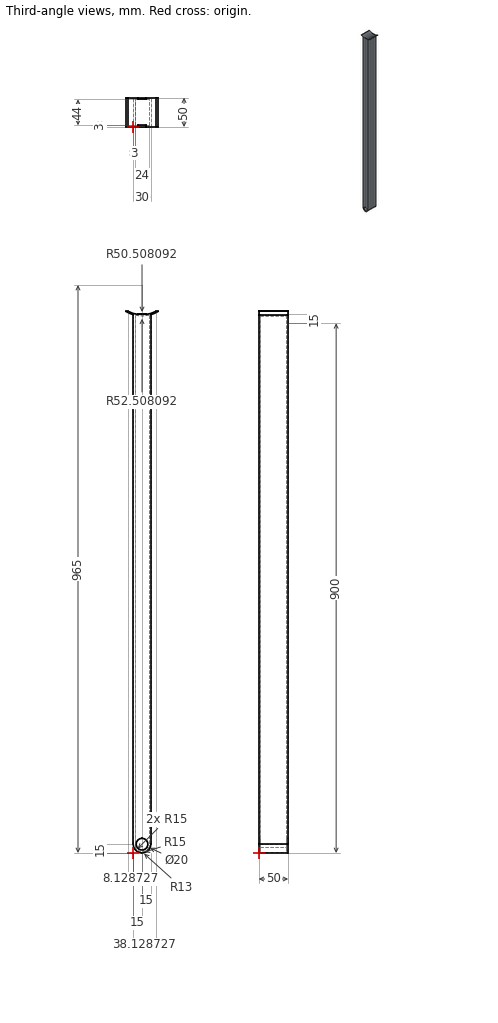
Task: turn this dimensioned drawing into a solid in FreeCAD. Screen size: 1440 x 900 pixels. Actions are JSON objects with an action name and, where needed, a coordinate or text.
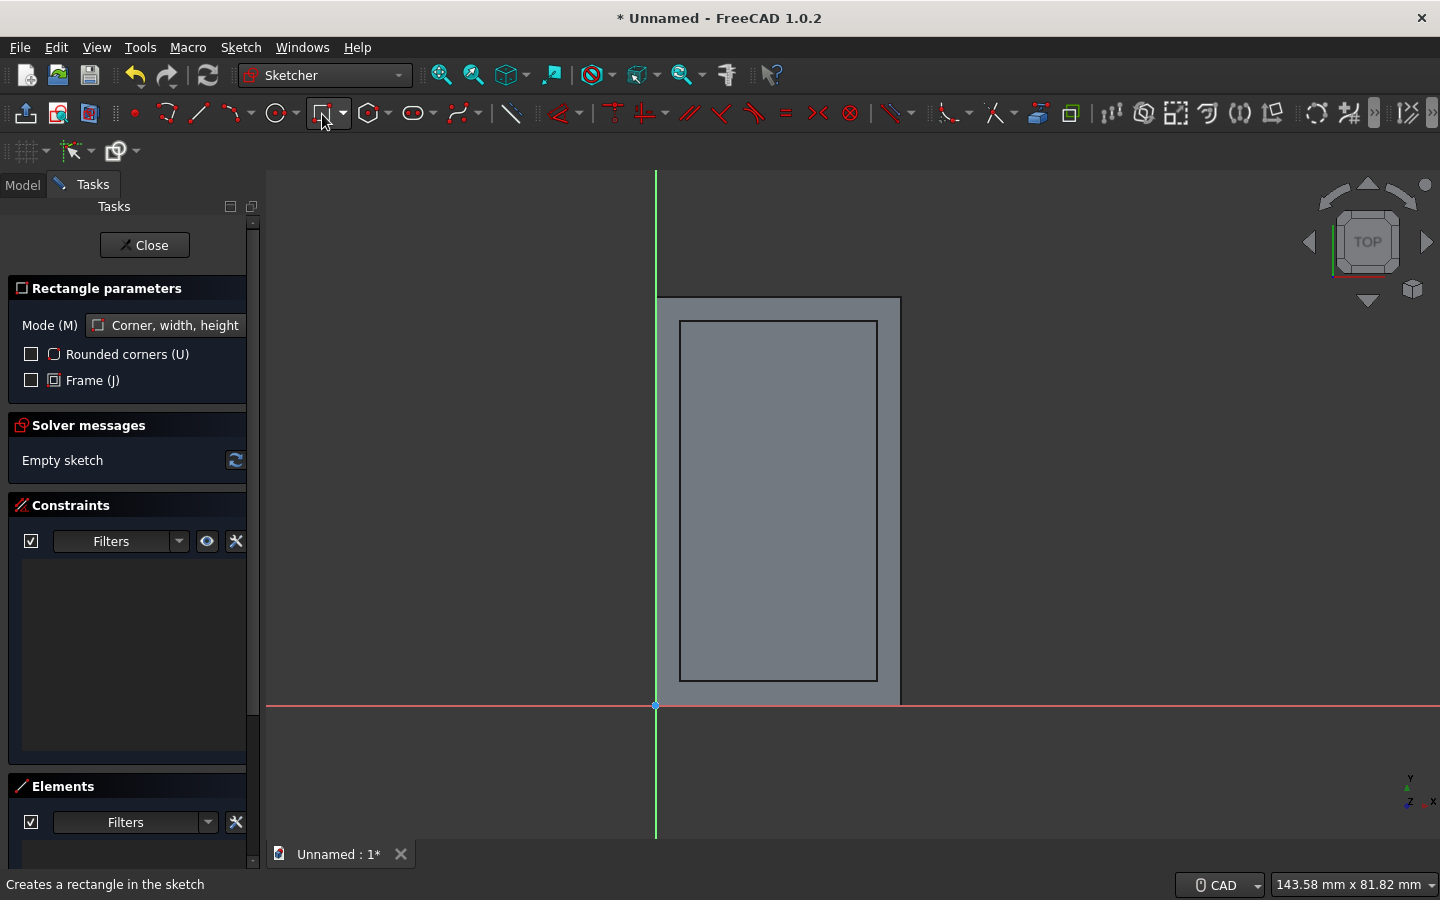
{"action": "left_click", "coordinate": [656, 706]}
{"action": "left_click", "coordinate": [901, 297]}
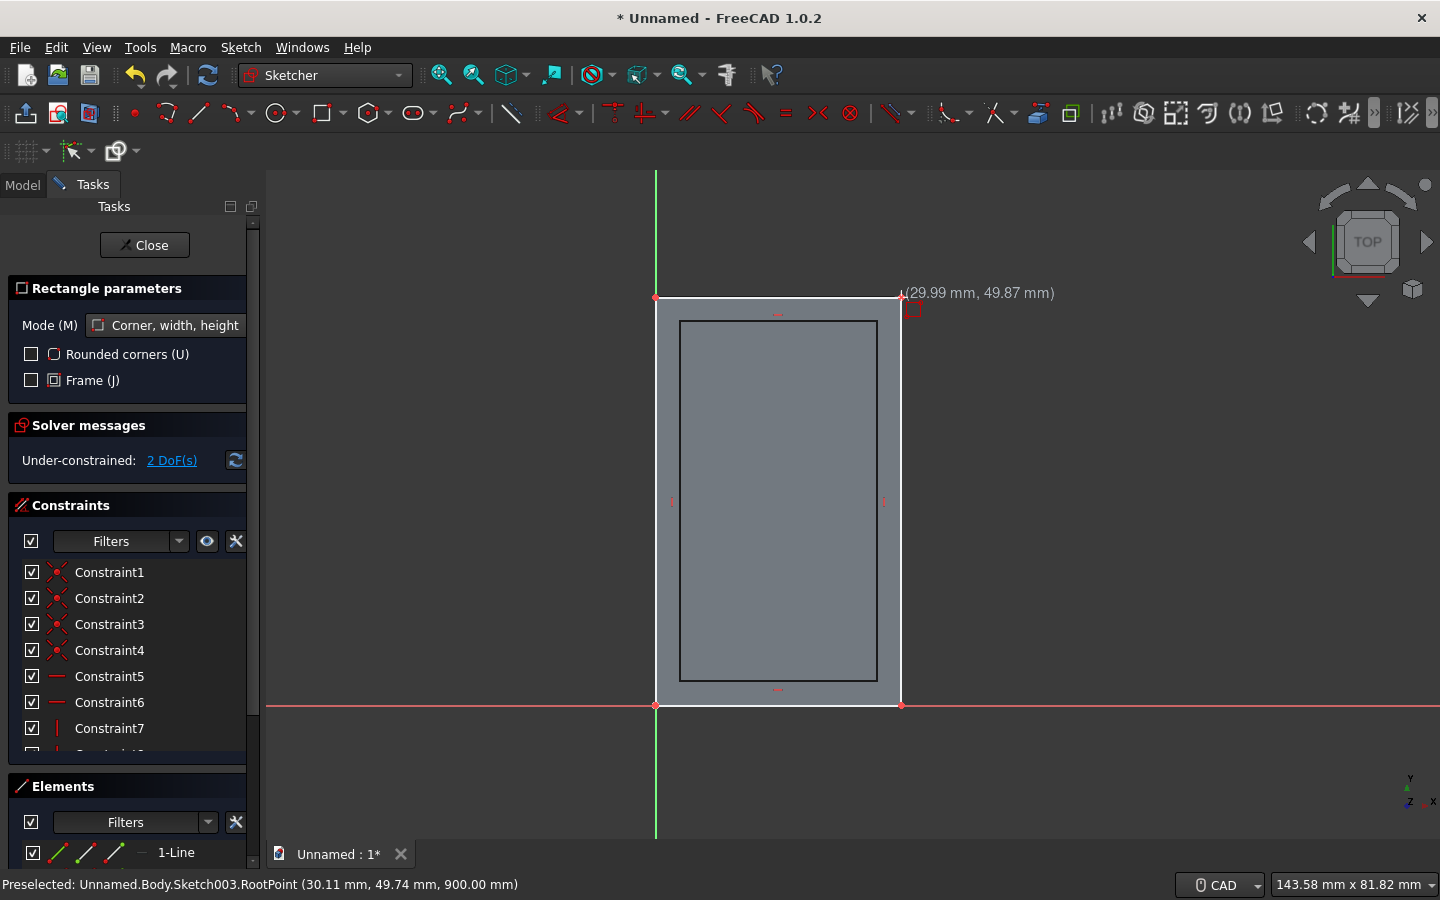
{"action": "left_click", "coordinate": [680, 321]}
{"action": "left_click", "coordinate": [877, 681]}
{"action": "key", "text": "Escape"}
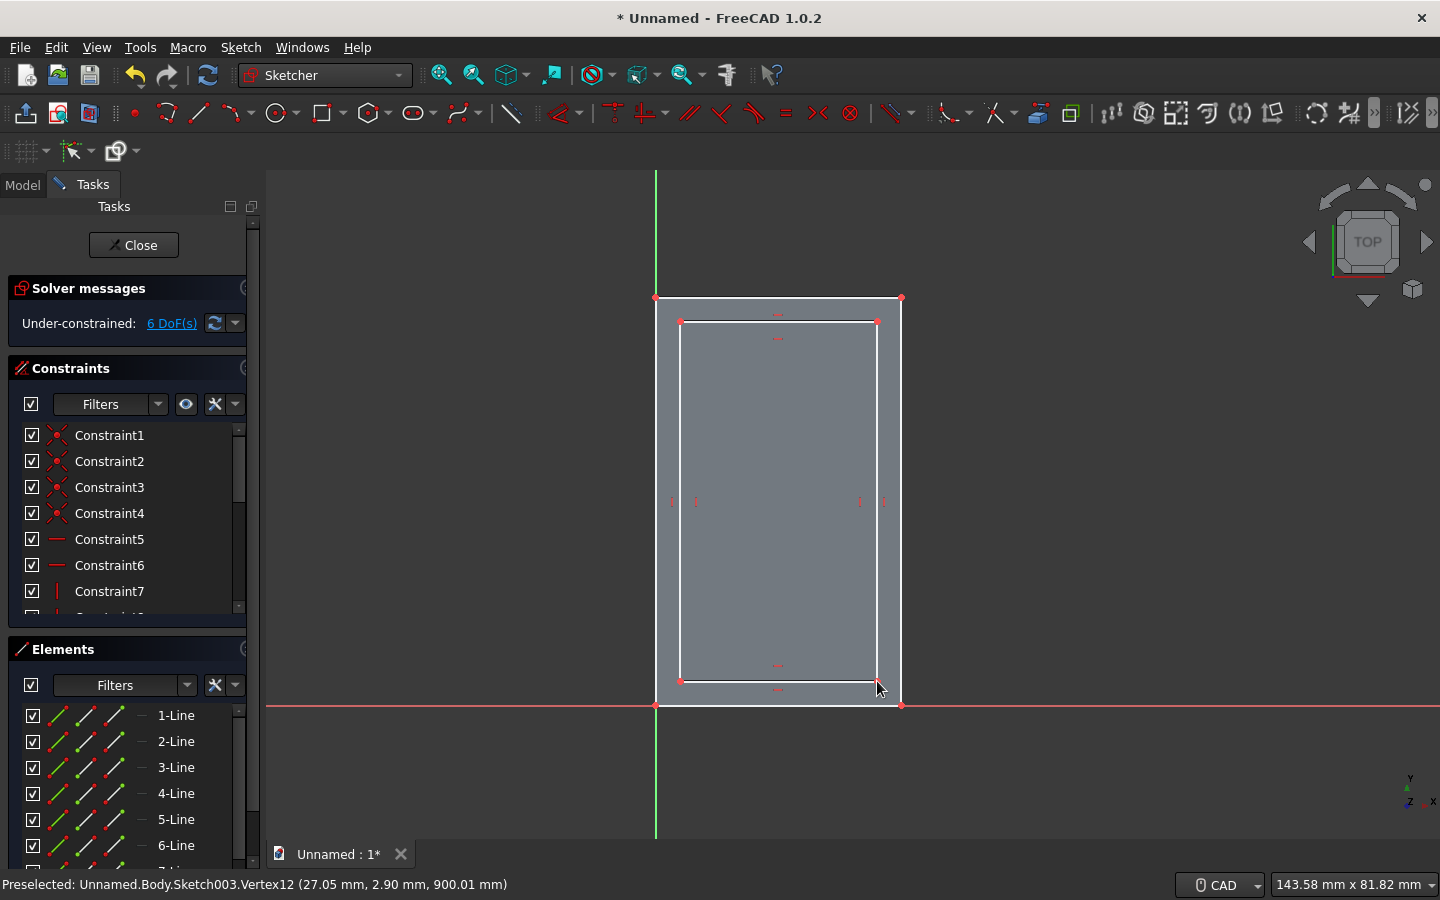
{"action": "left_click", "coordinate": [558, 114]}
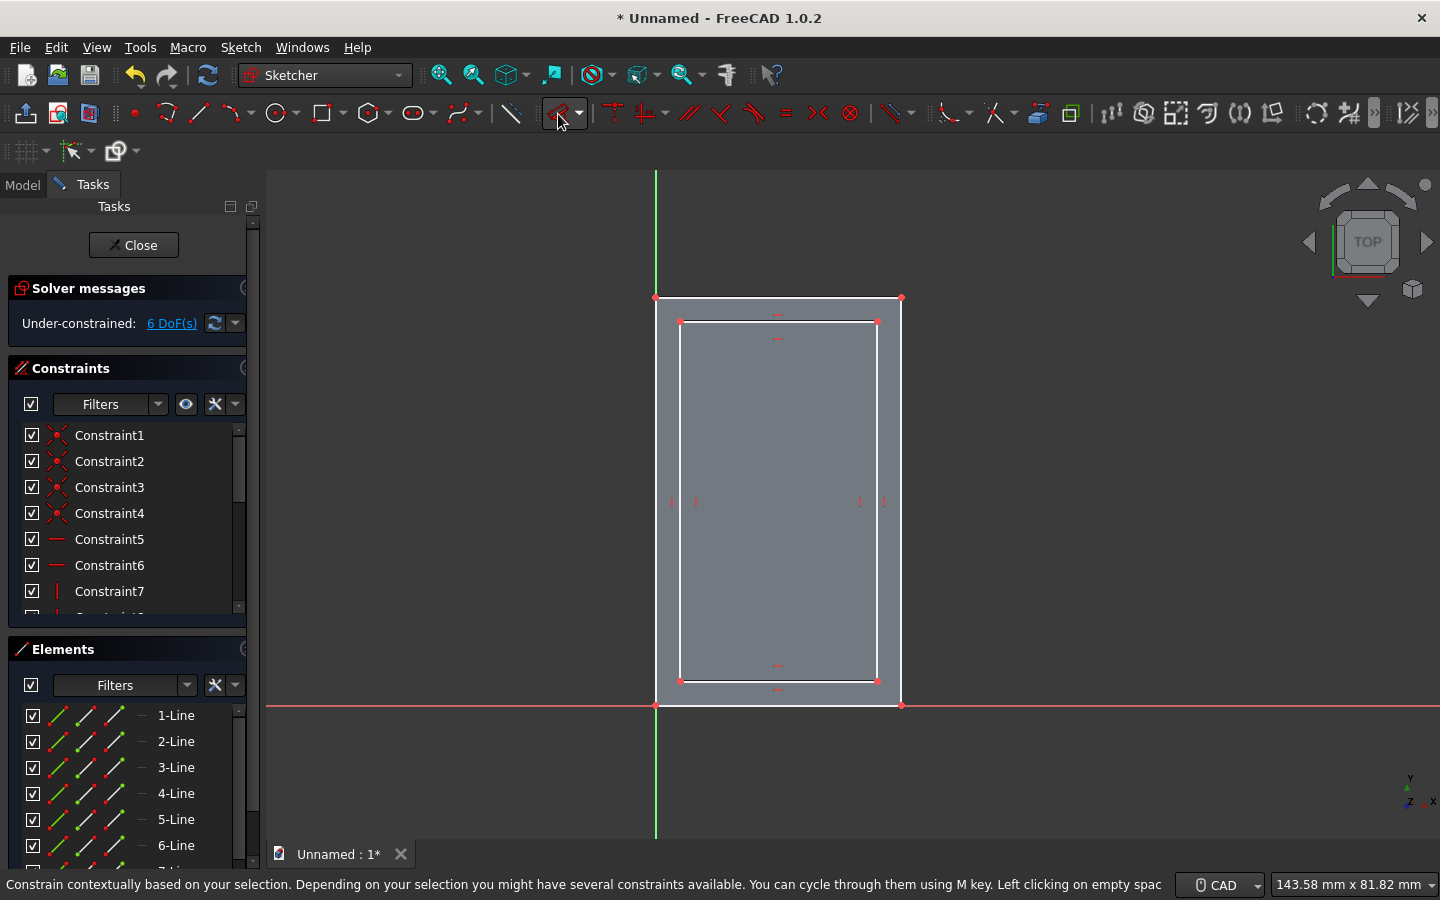
{"action": "left_click", "coordinate": [729, 706]}
{"action": "left_click", "coordinate": [778, 740]}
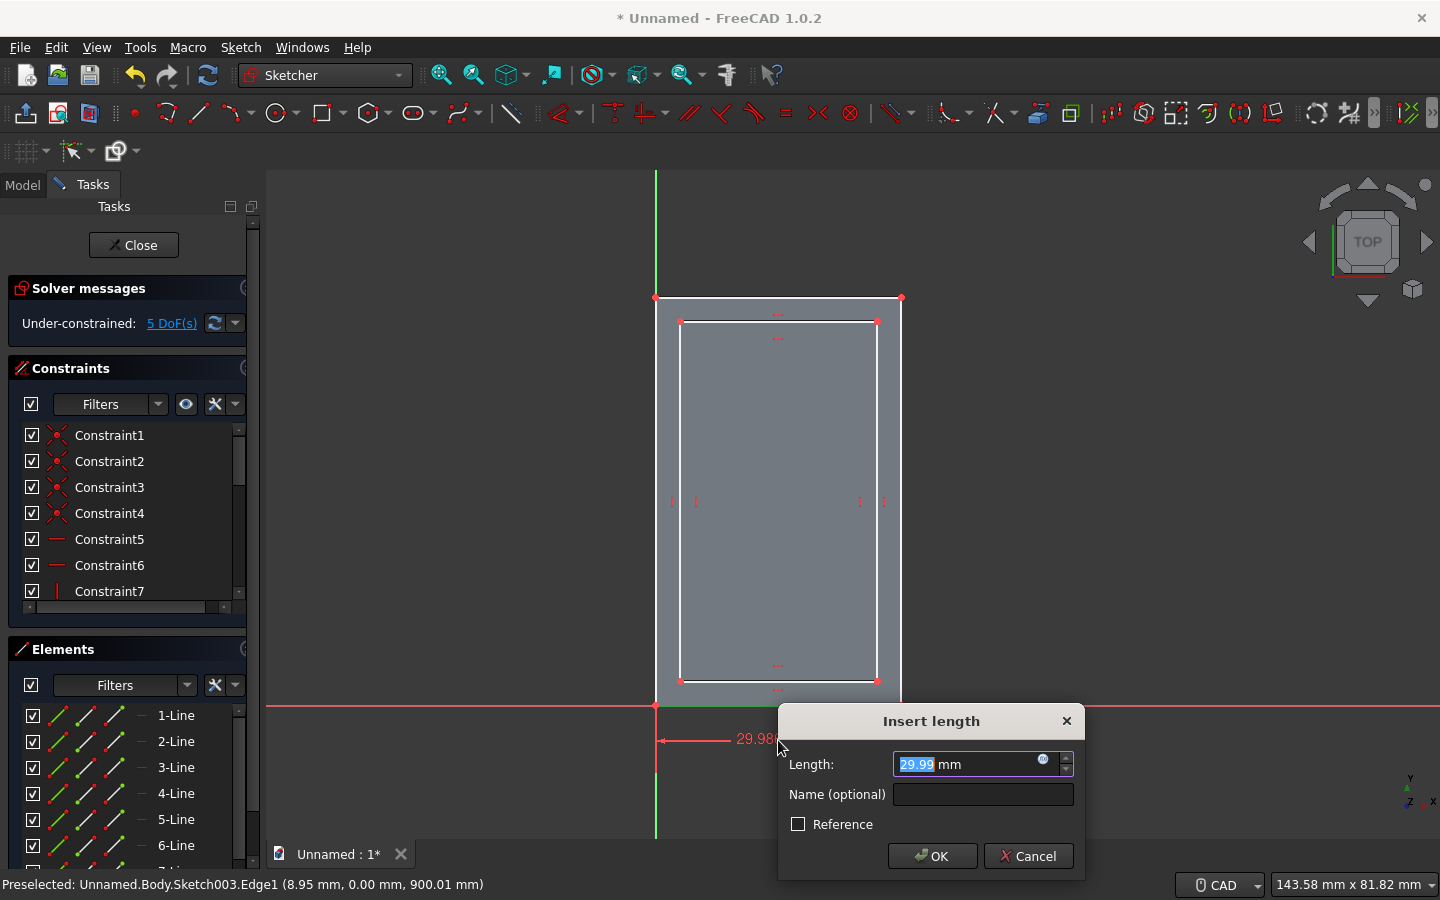
{"action": "type", "text": "30"}
{"action": "key", "text": "Return"}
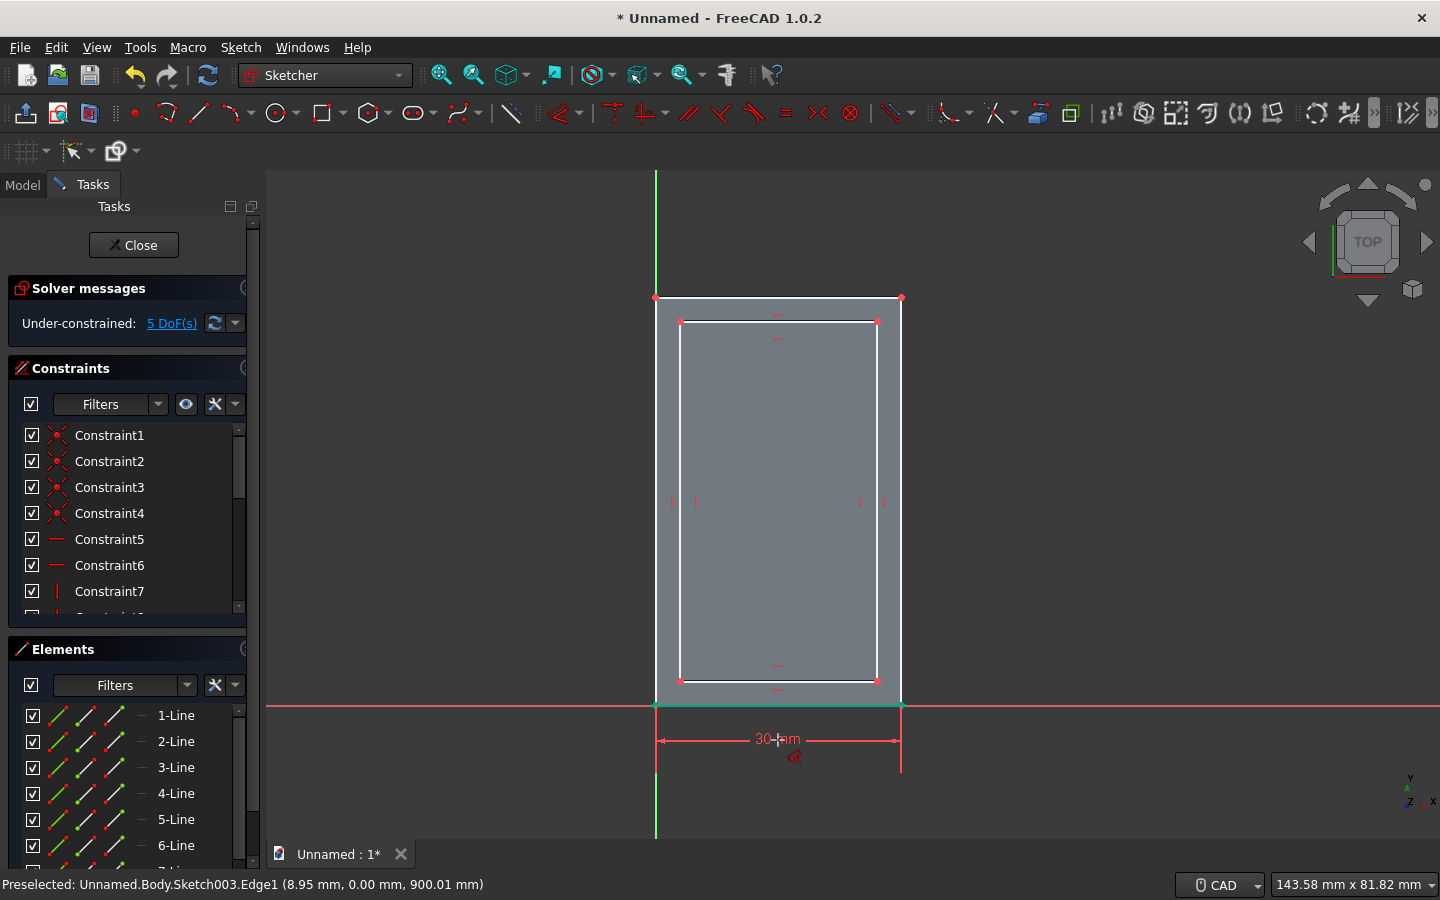
{"action": "left_click", "coordinate": [901, 583]}
{"action": "left_click", "coordinate": [935, 502]}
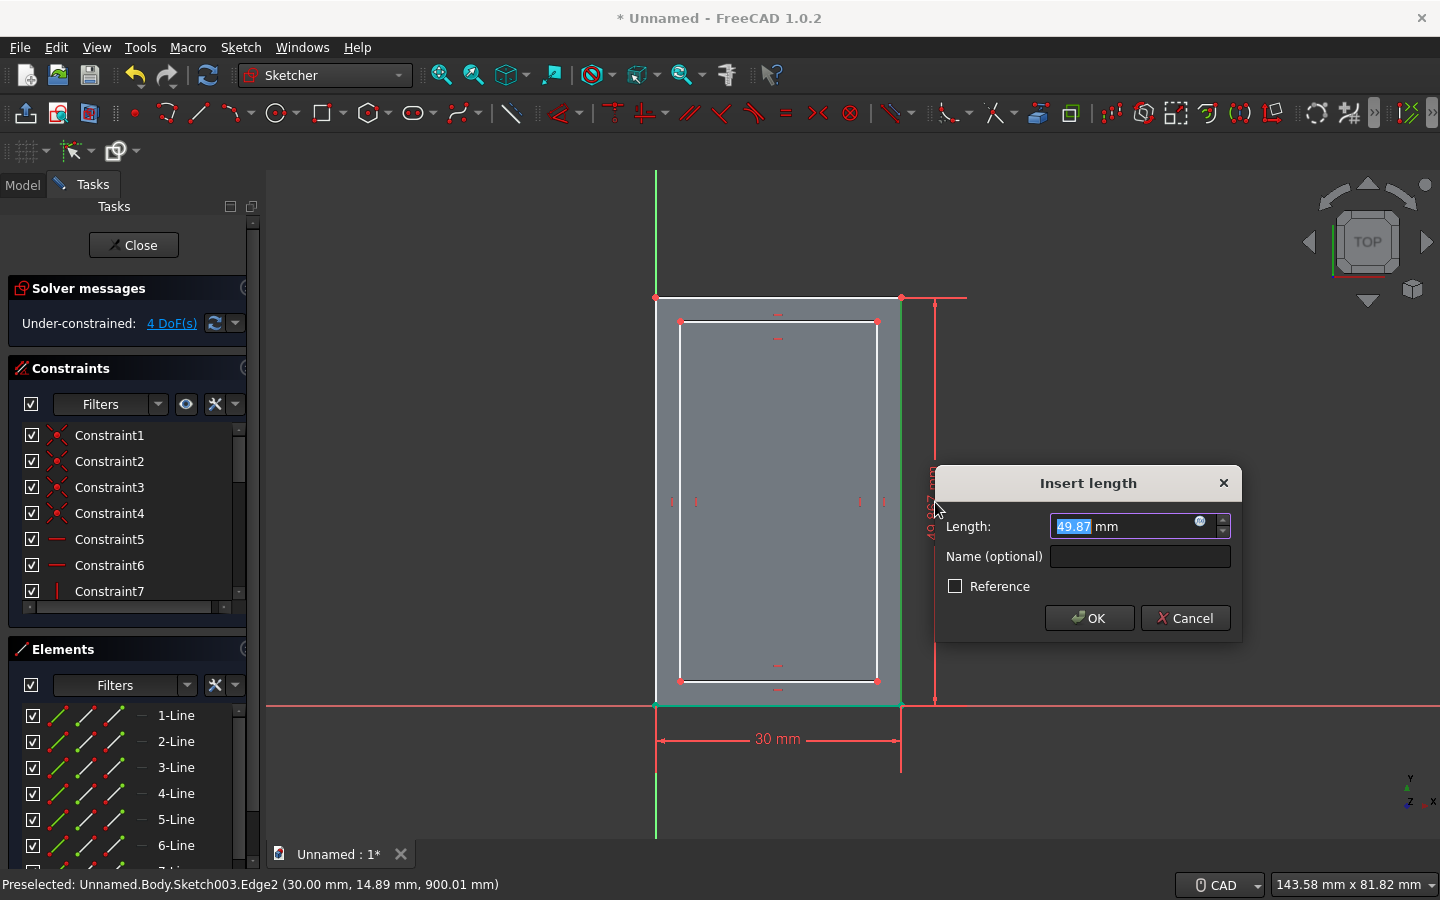
{"action": "type", "text": "50"}
{"action": "key", "text": "Return"}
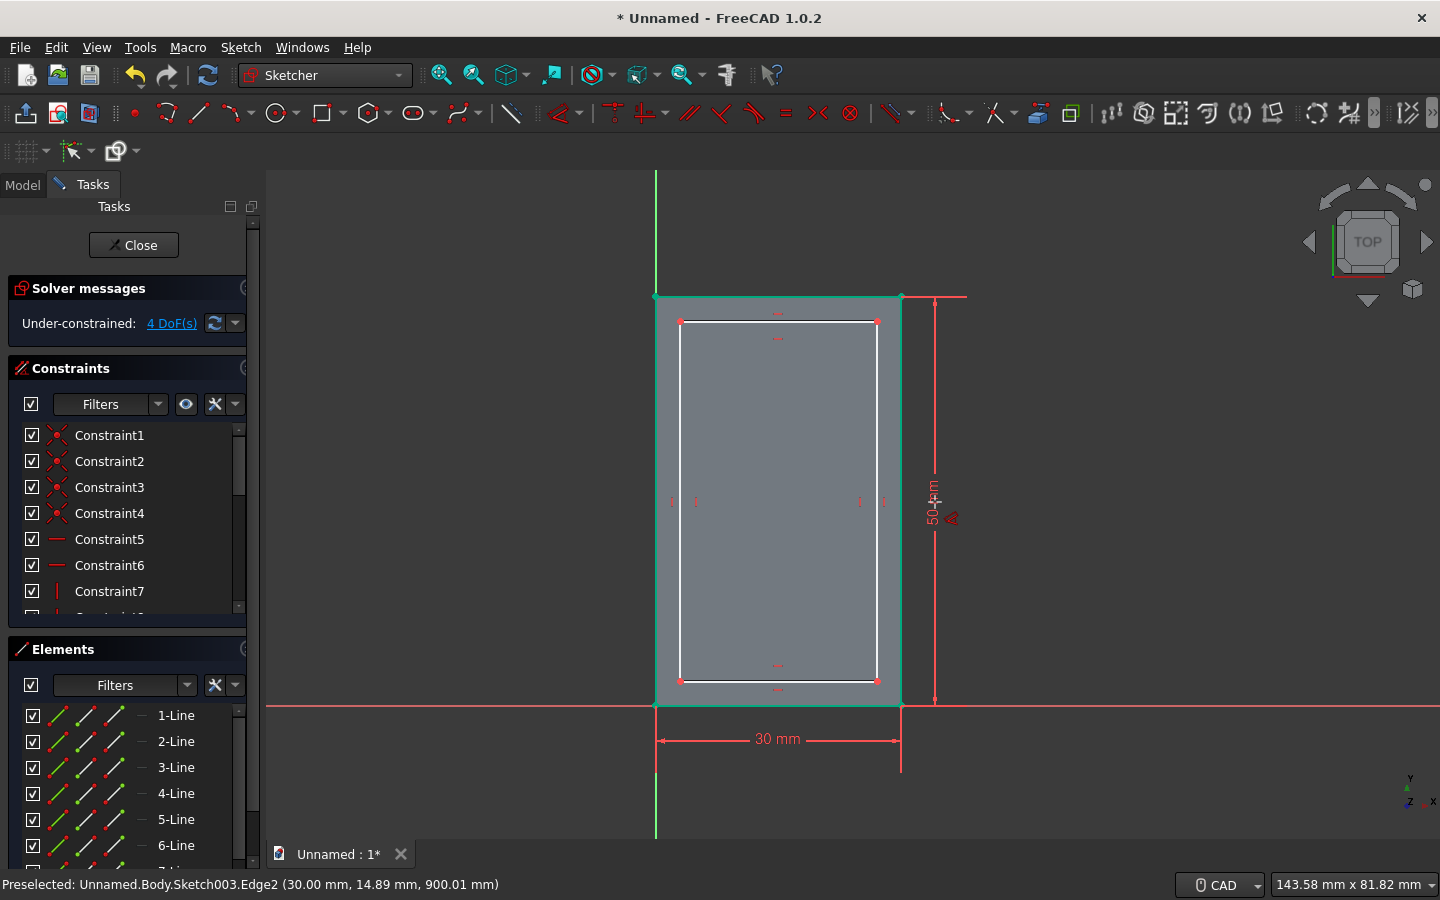
{"action": "left_click", "coordinate": [680, 430]}
{"action": "left_click", "coordinate": [714, 502]}